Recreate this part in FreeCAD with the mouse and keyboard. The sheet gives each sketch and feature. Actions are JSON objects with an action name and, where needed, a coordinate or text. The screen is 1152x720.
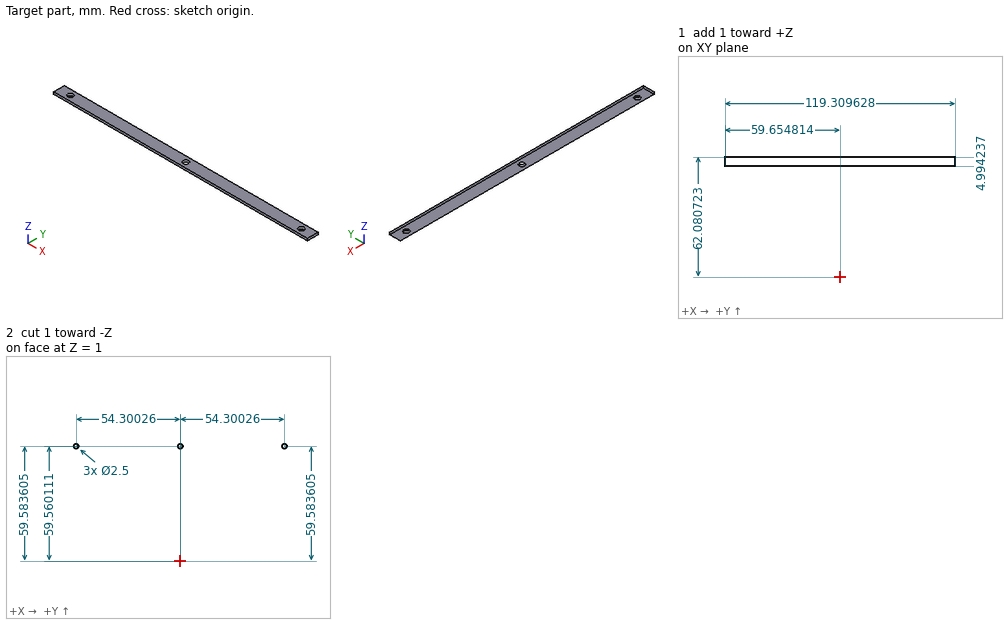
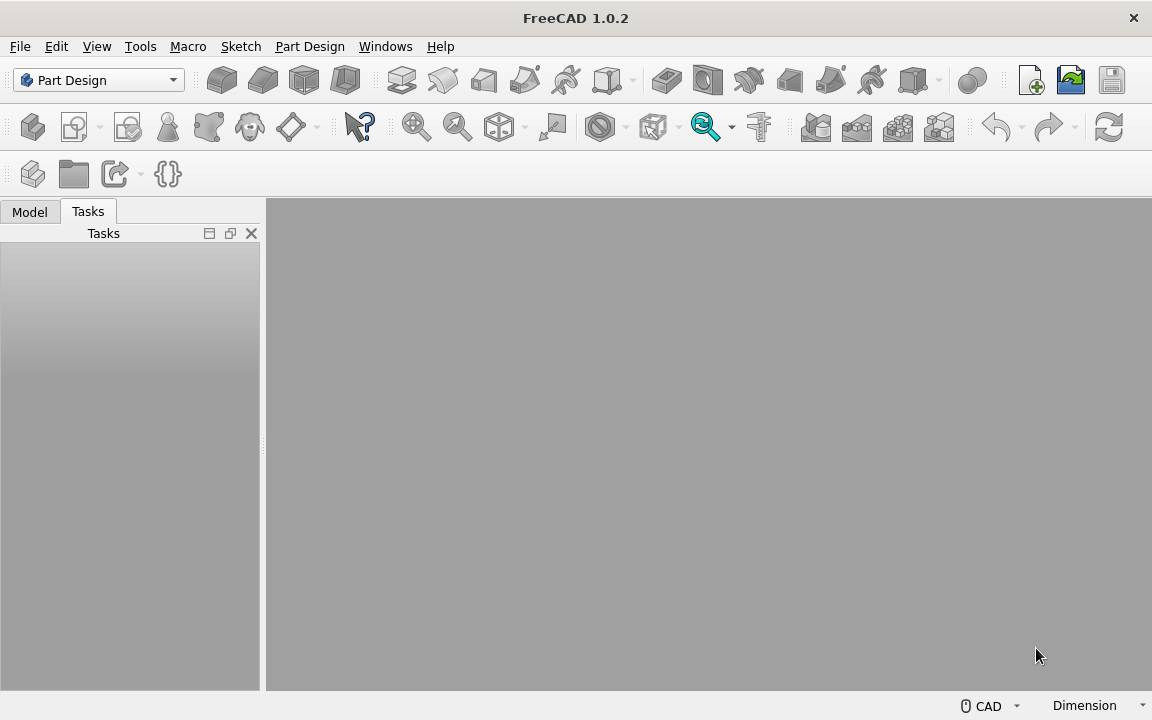
{"action": "key", "text": "ctrl+n"}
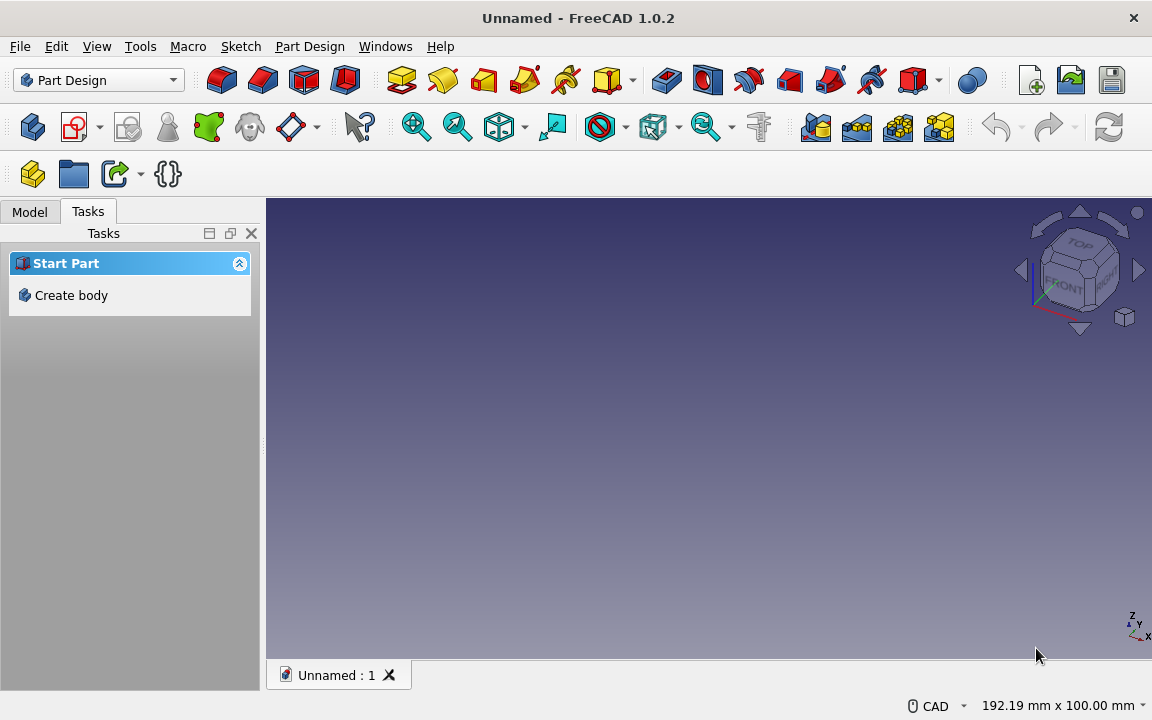
{"action": "left_click", "coordinate": [74, 128]}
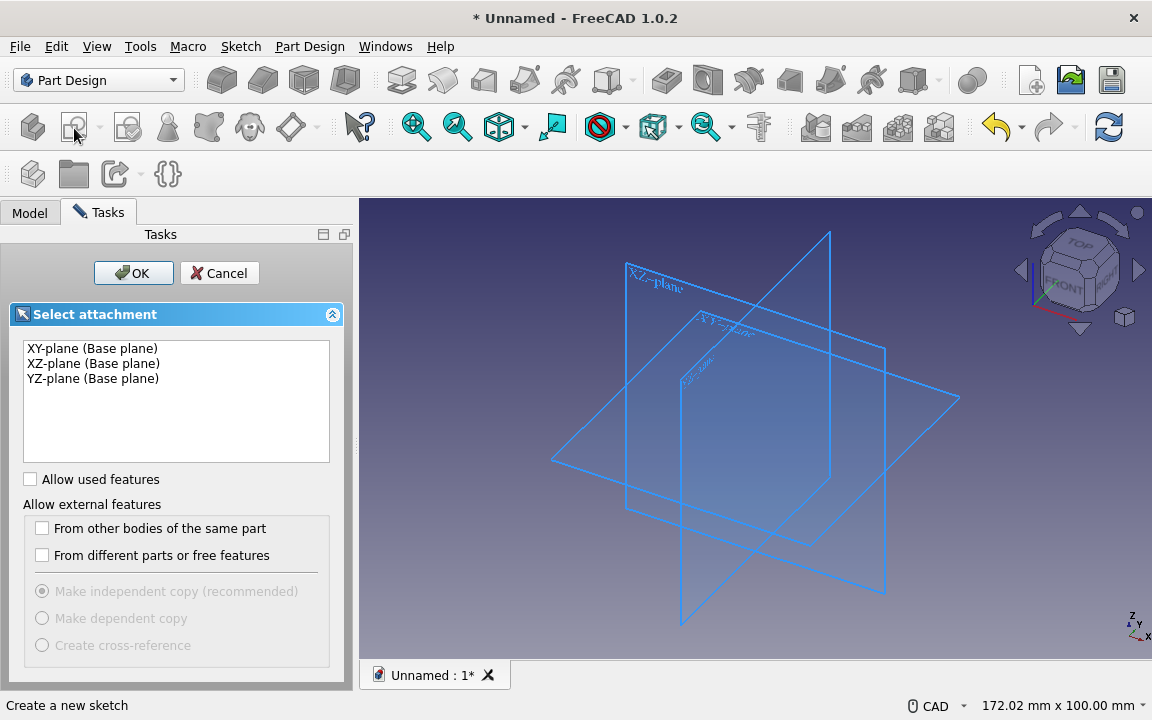
{"action": "left_click", "coordinate": [84, 348]}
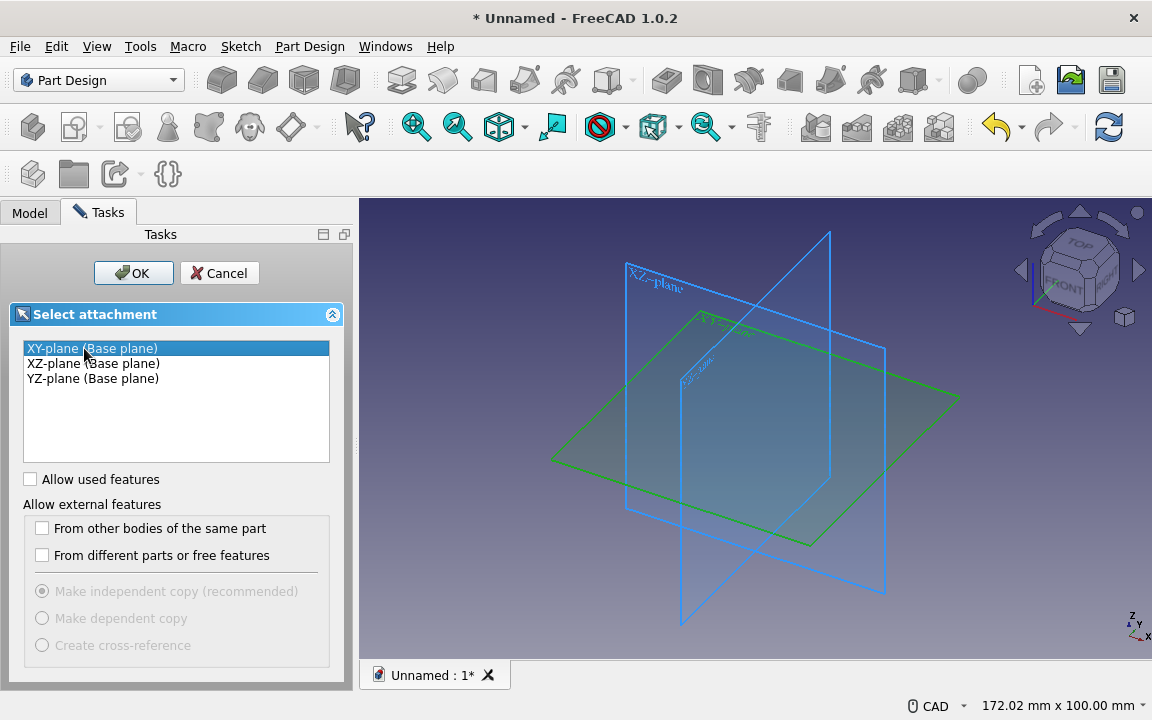
{"action": "left_click", "coordinate": [134, 273]}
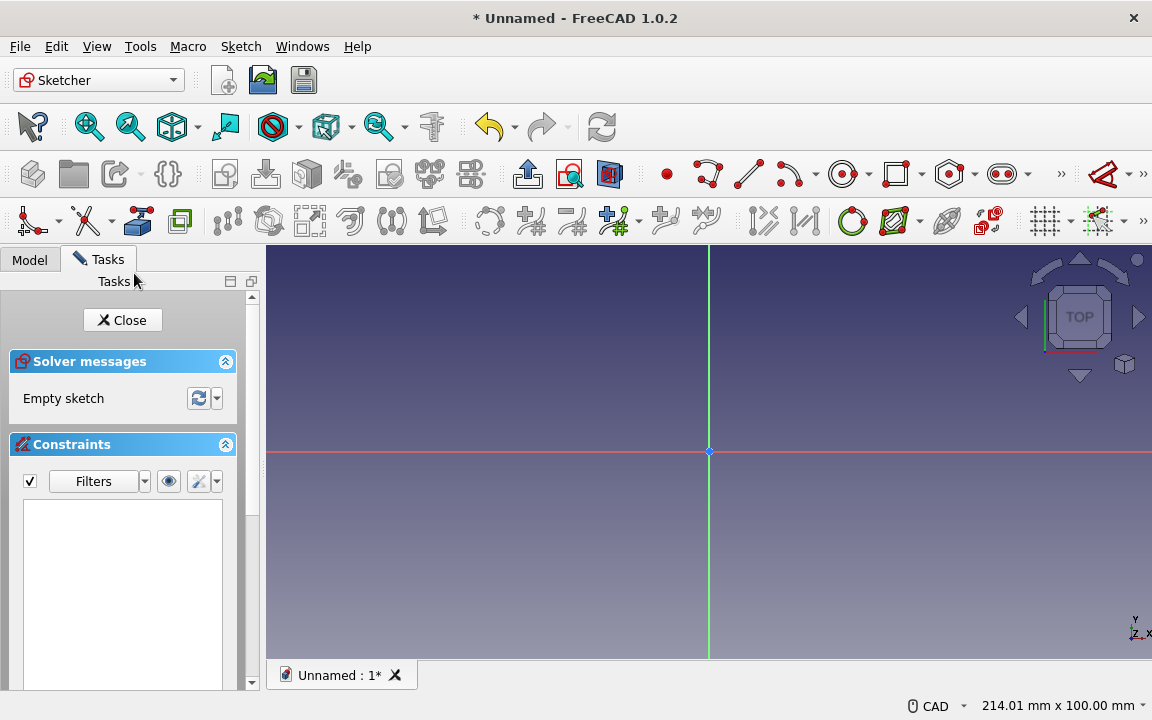
{"action": "scroll", "coordinate": [501, 631], "scroll_direction": "down", "scroll_amount": 2}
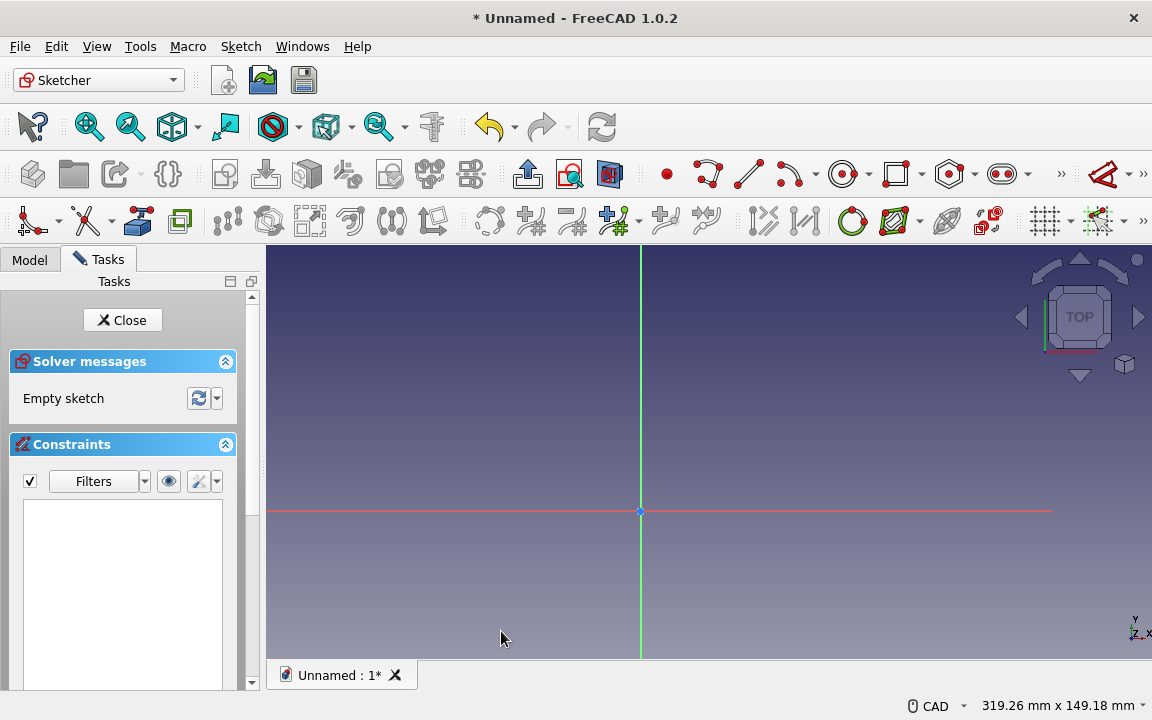
{"action": "scroll", "coordinate": [641, 371], "scroll_direction": "up", "scroll_amount": 2}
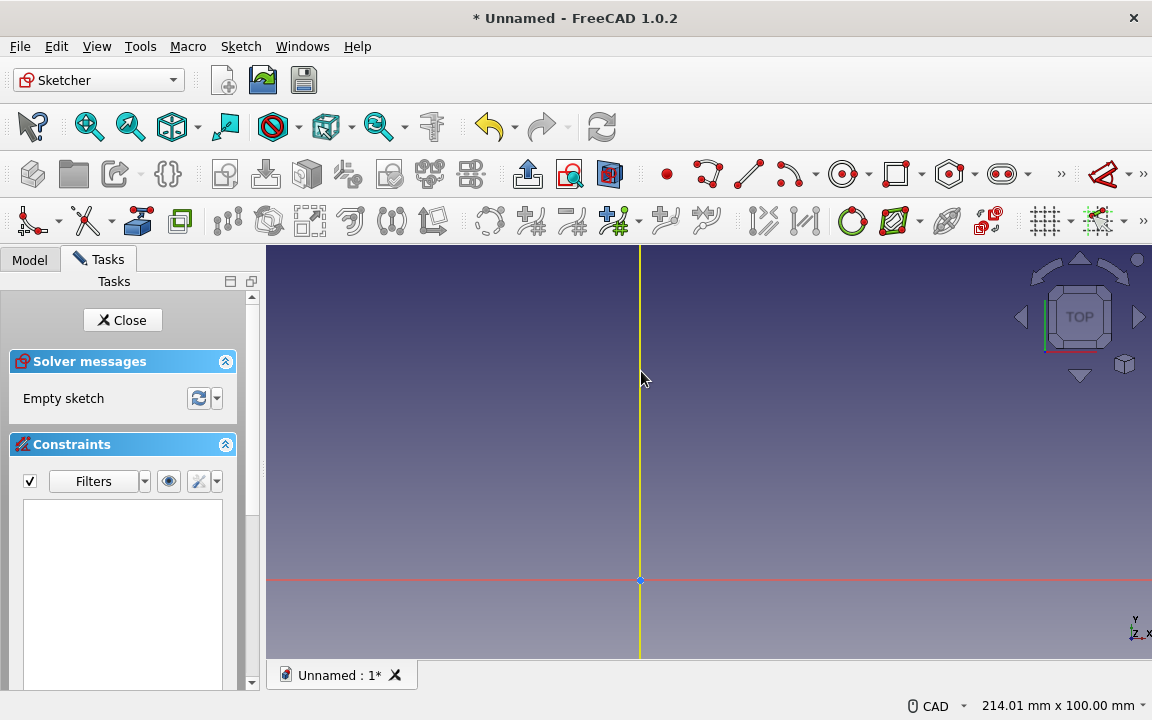
{"action": "key", "text": "g r"}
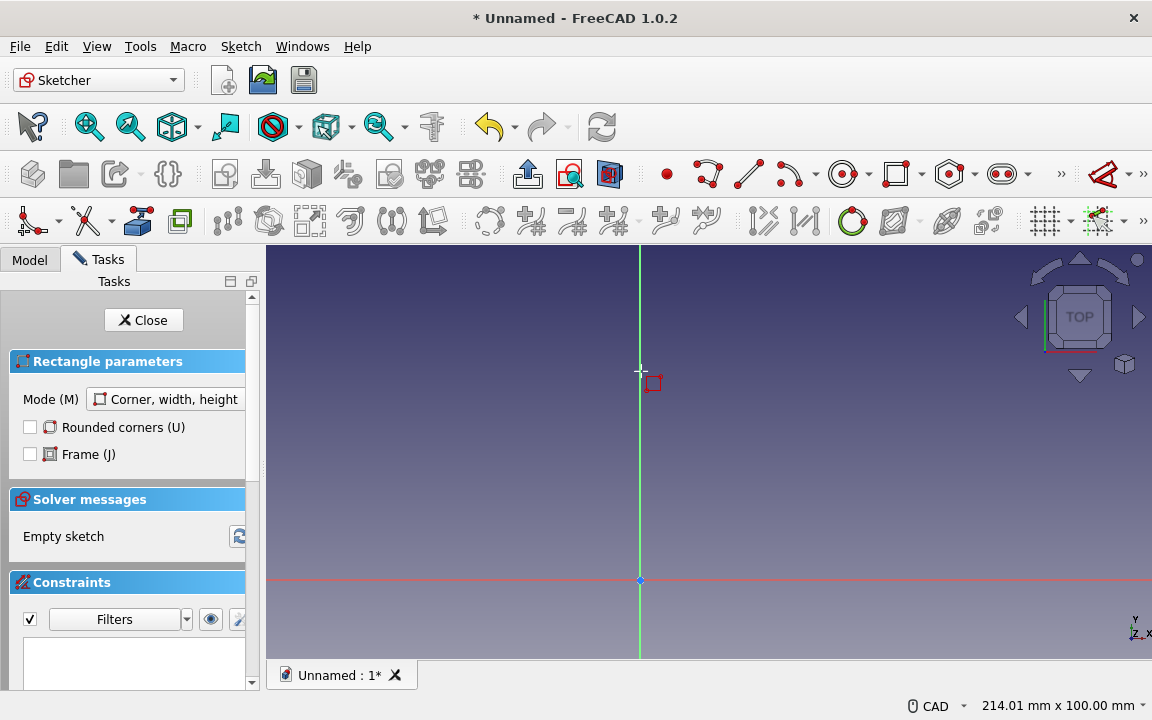
{"action": "left_click", "coordinate": [393, 323]}
{"action": "mouse_move", "coordinate": [887, 344]}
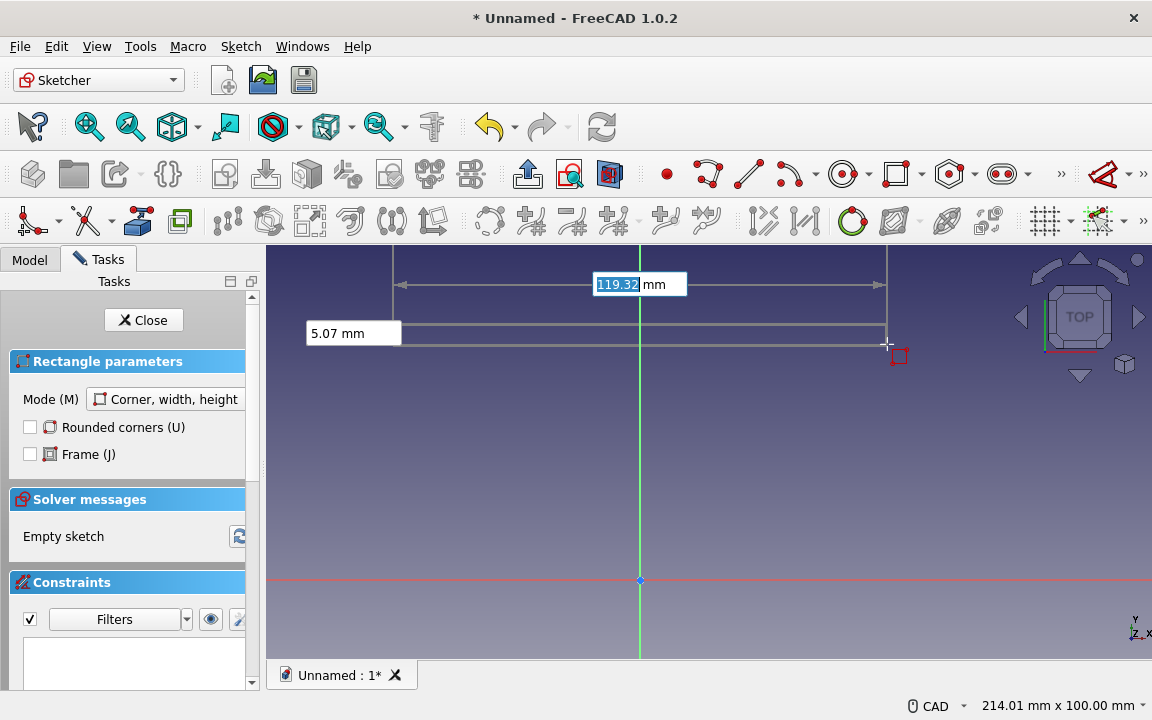
{"action": "type", "text": "119.309628"}
{"action": "key", "text": "Tab"}
{"action": "type", "text": "4.994237"}
{"action": "key", "text": "Return"}
{"action": "key", "text": "Escape"}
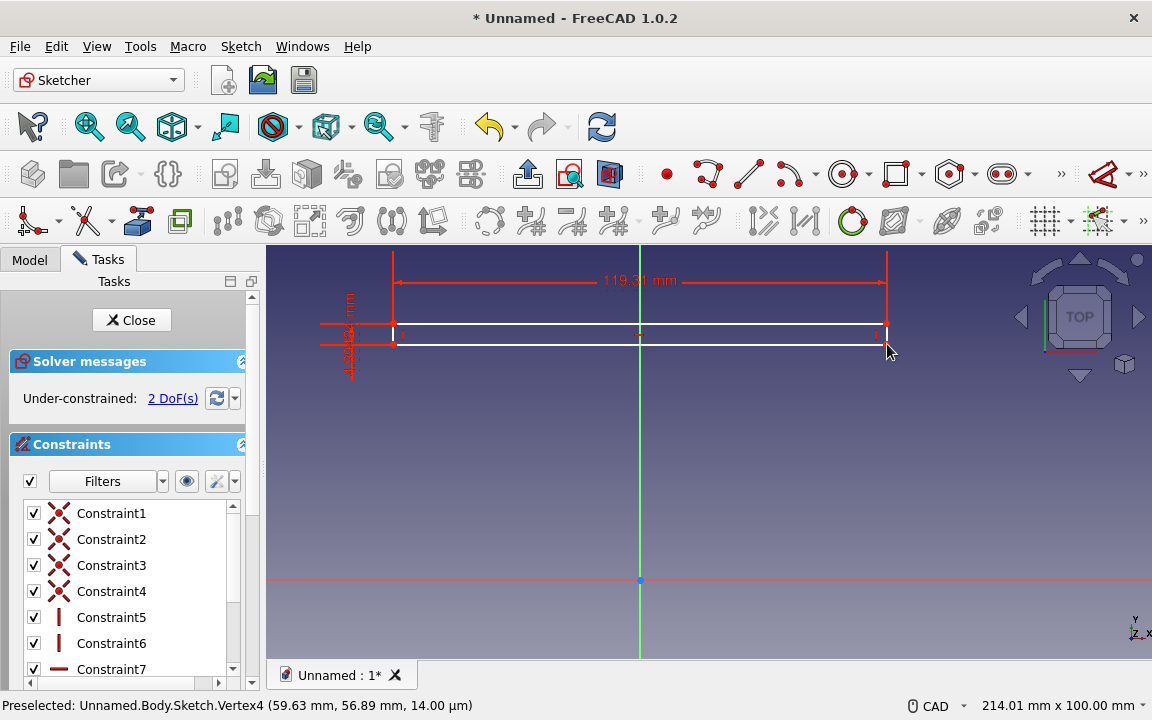
{"action": "left_click", "coordinate": [1102, 174]}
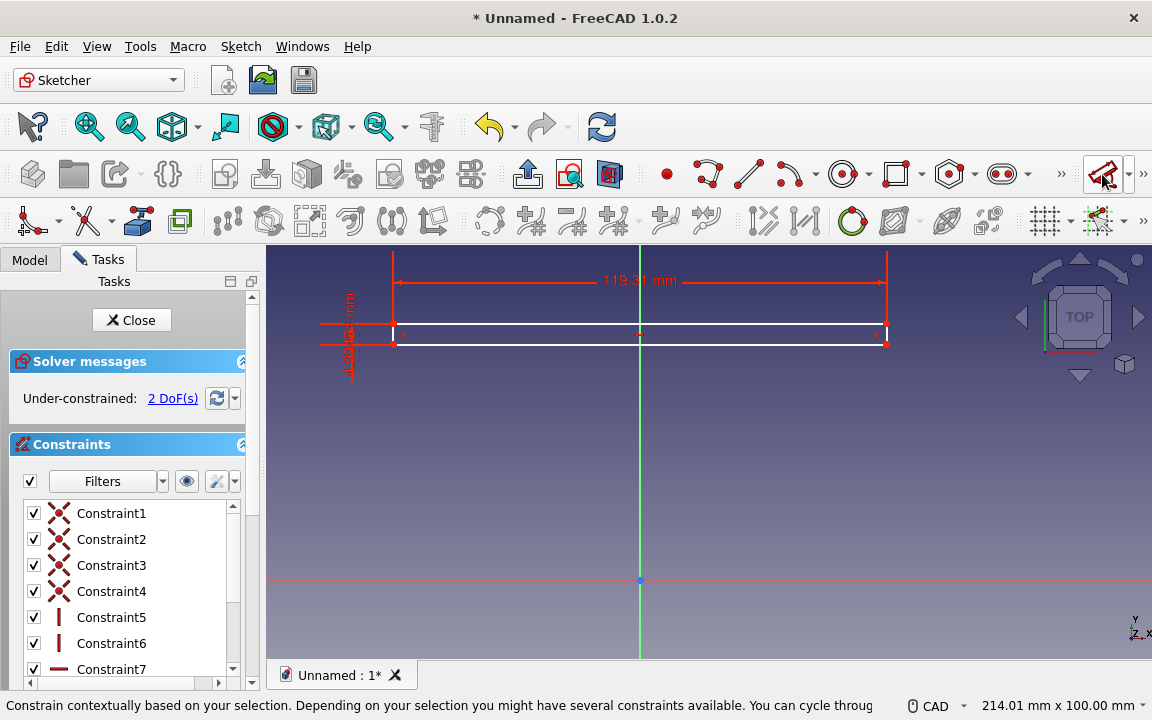
{"action": "left_click", "coordinate": [393, 324]}
{"action": "left_click", "coordinate": [517, 614]}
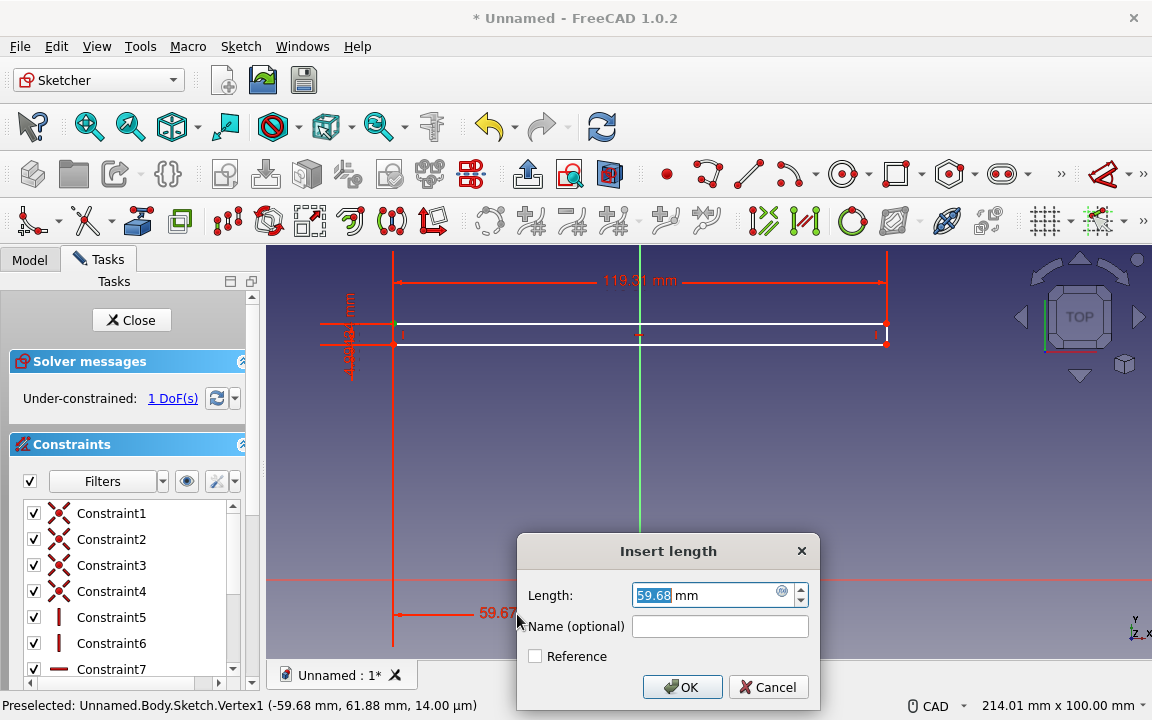
{"action": "type", "text": "59.654814"}
{"action": "key", "text": "Return"}